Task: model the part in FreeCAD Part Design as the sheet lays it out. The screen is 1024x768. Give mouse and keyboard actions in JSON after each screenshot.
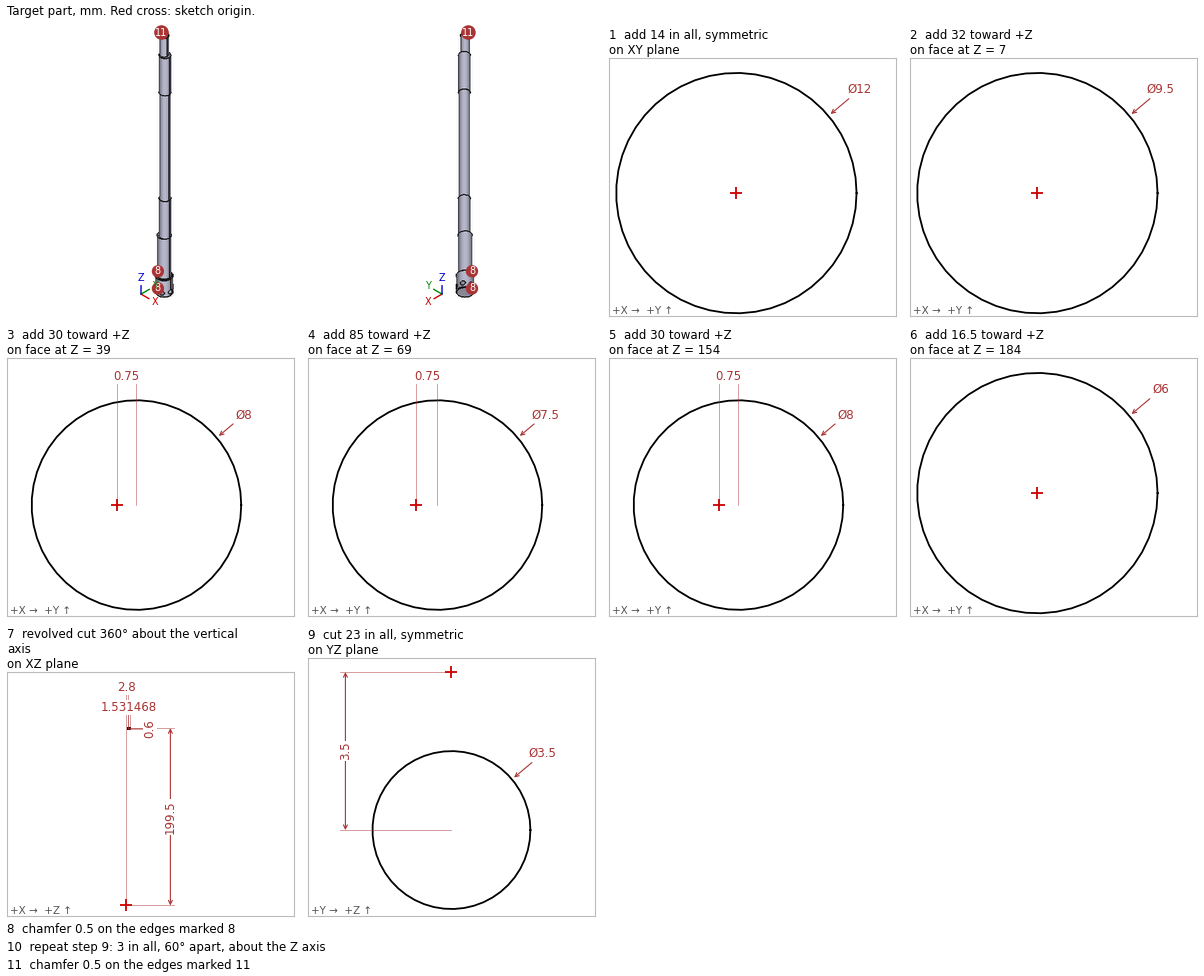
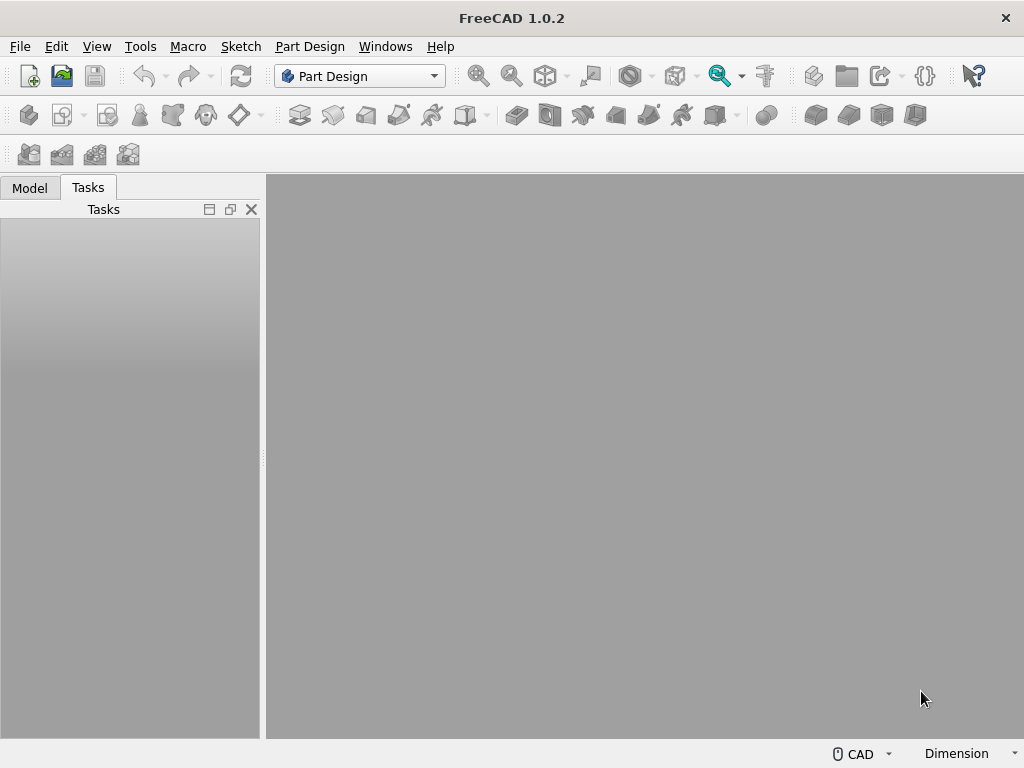
{"action": "left_click", "coordinate": [29, 76]}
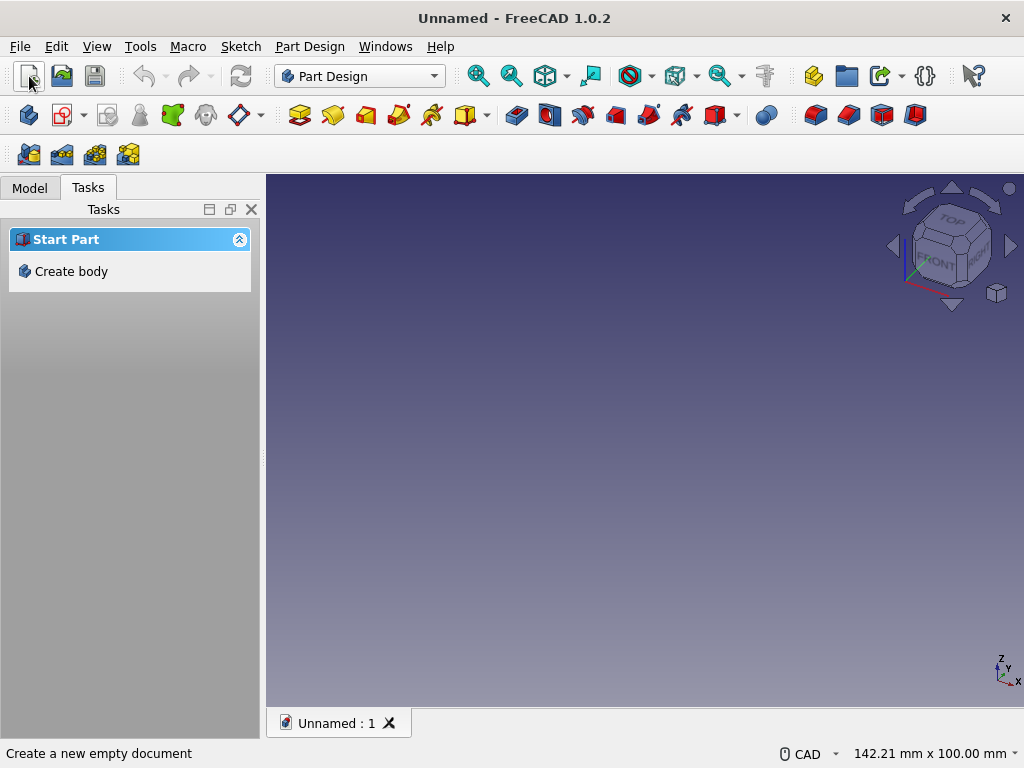
{"action": "left_click", "coordinate": [62, 116]}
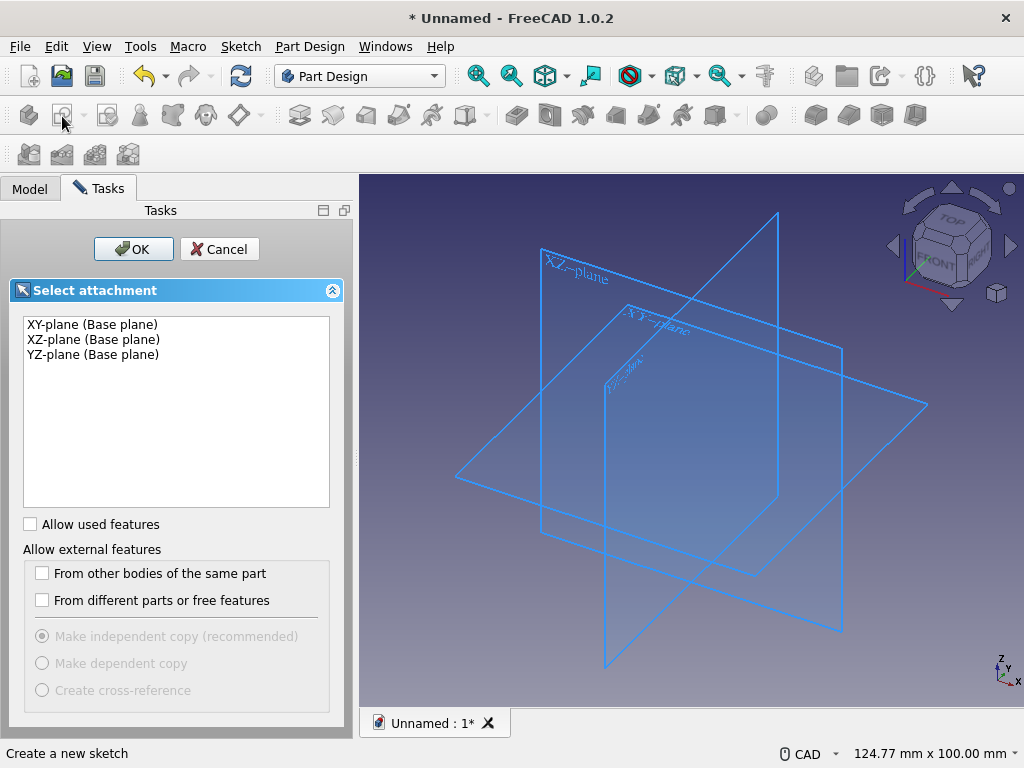
{"action": "left_click", "coordinate": [84, 324]}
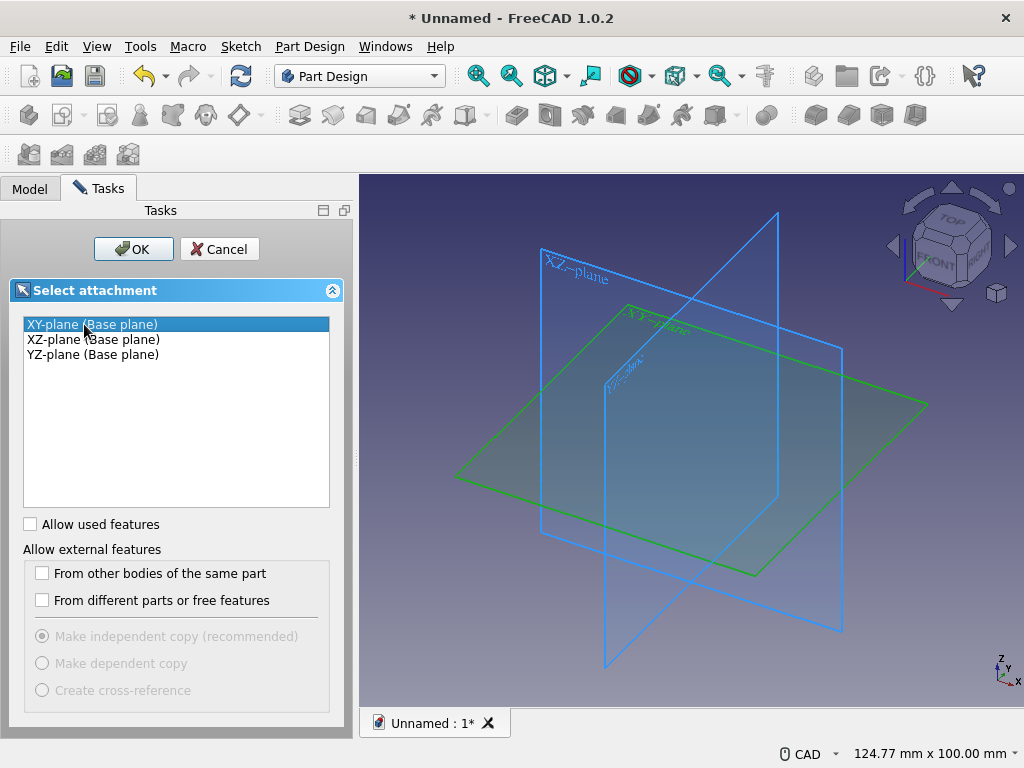
{"action": "left_click", "coordinate": [134, 249]}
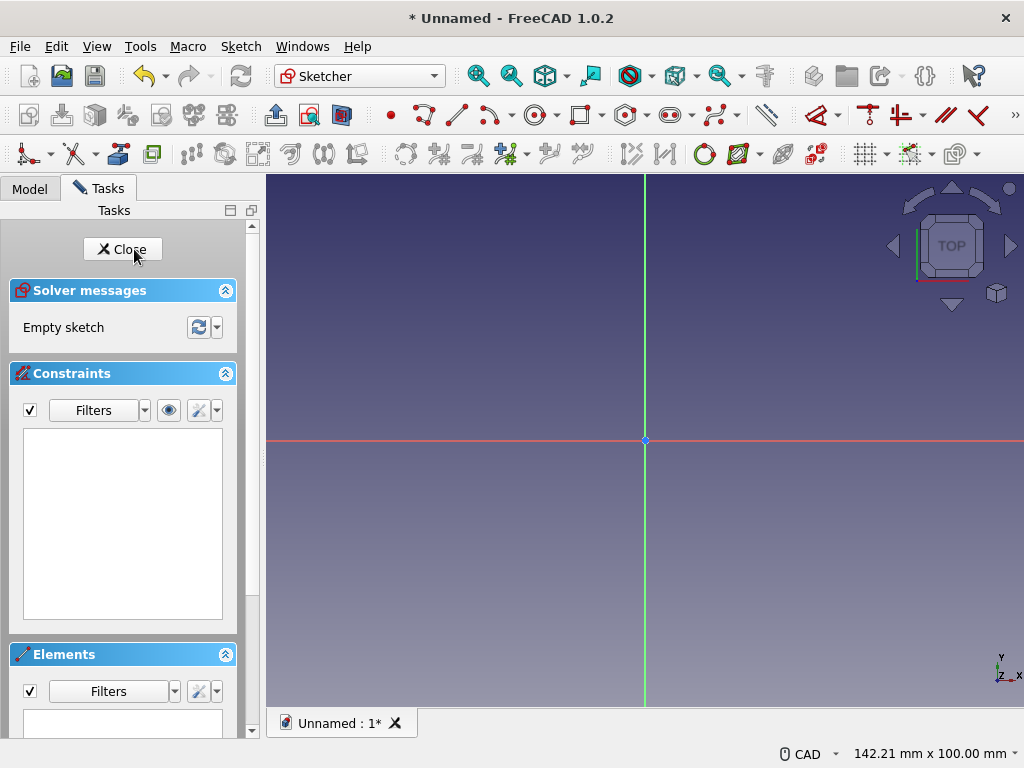
{"action": "scroll", "coordinate": [662, 440], "scroll_direction": "up", "scroll_amount": 8}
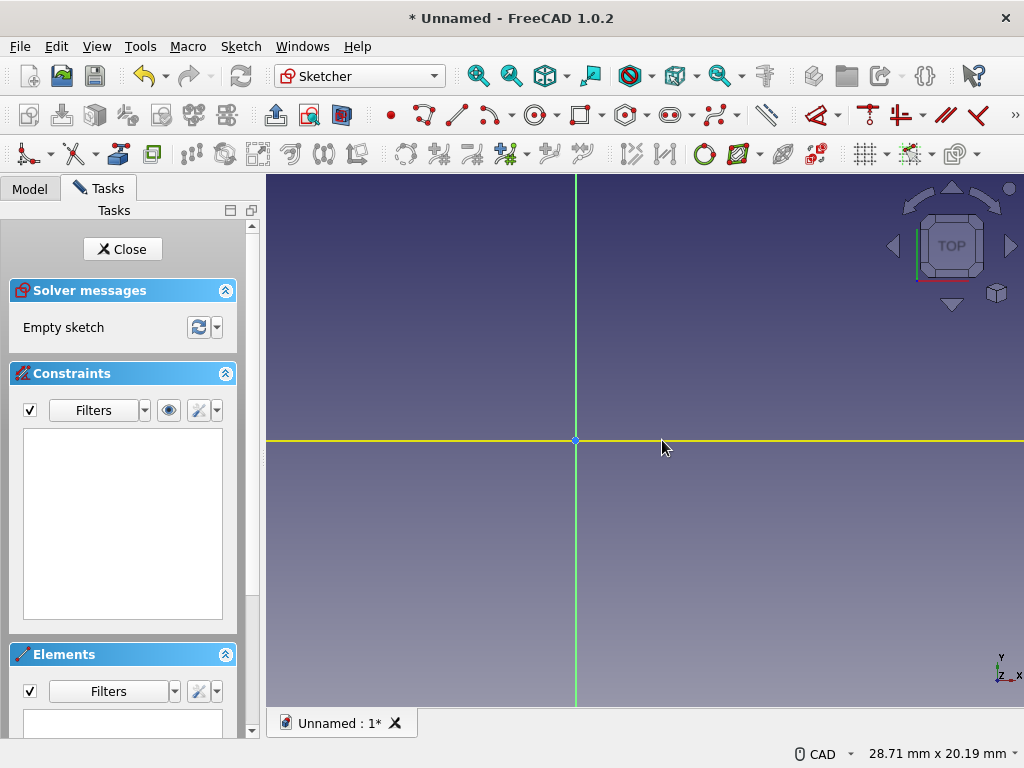
{"action": "left_click", "coordinate": [534, 116]}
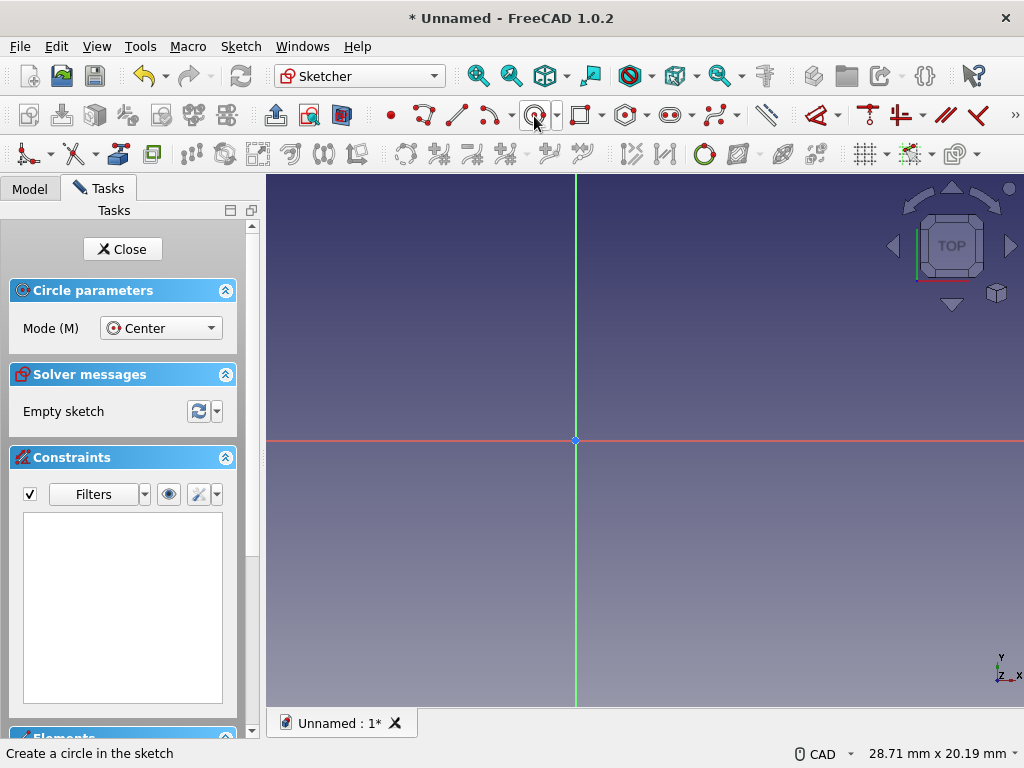
{"action": "left_click", "coordinate": [576, 440]}
{"action": "left_click", "coordinate": [688, 328]}
{"action": "key", "text": "Escape"}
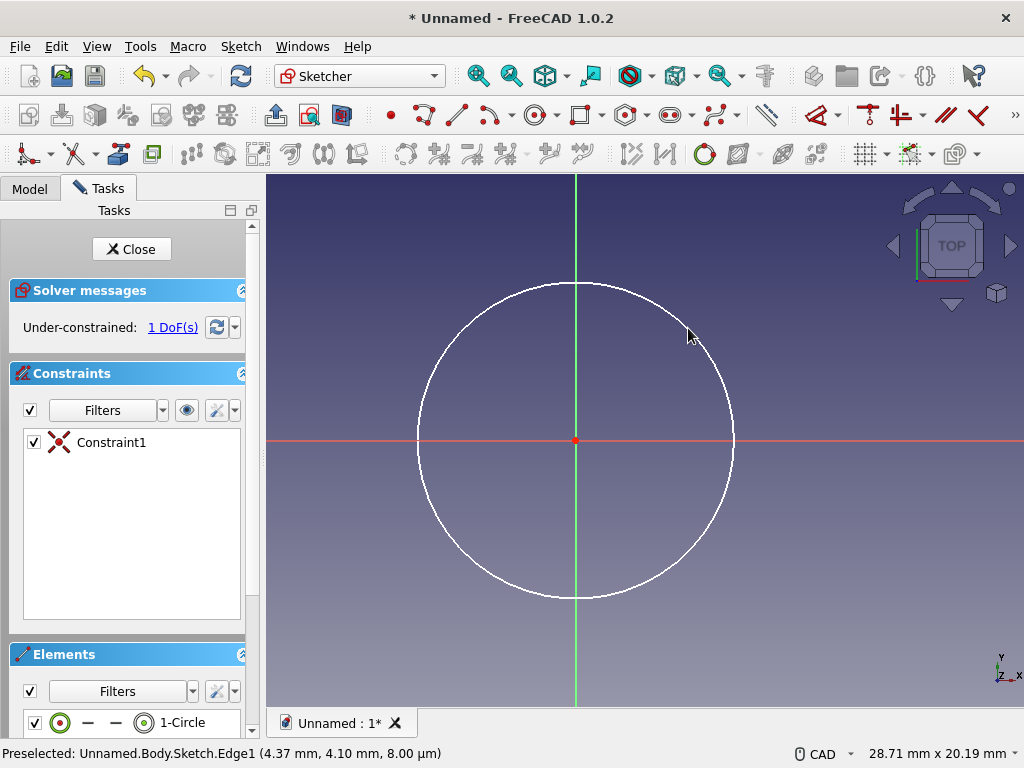
{"action": "left_click", "coordinate": [687, 328]}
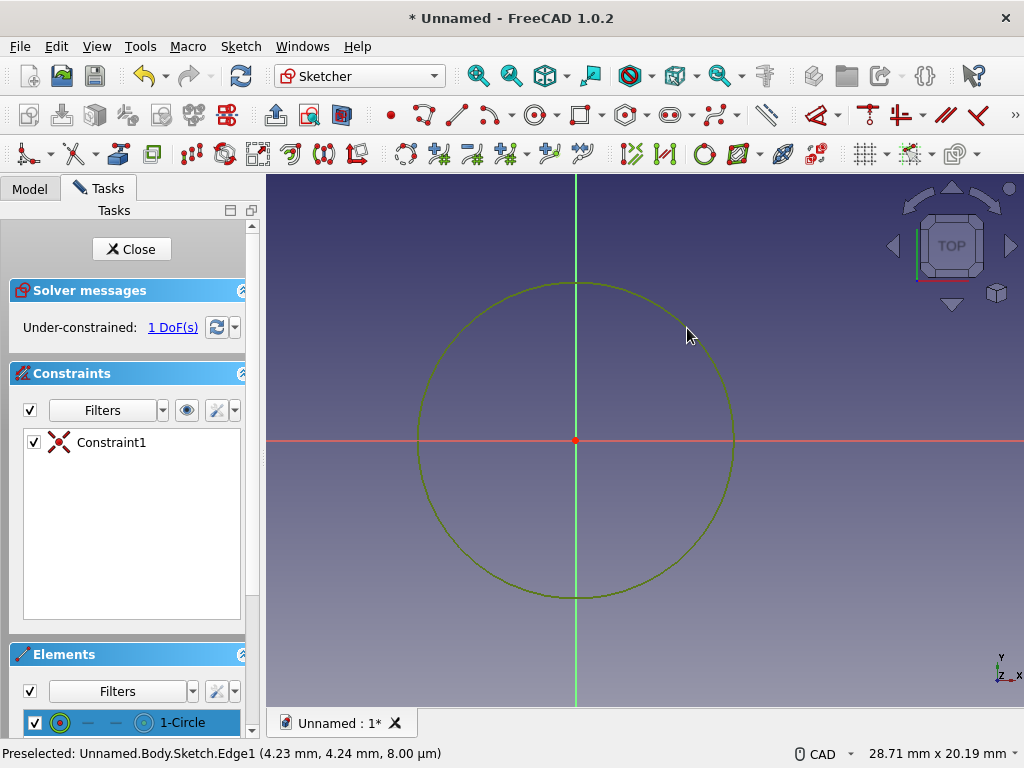
{"action": "left_click", "coordinate": [838, 116]}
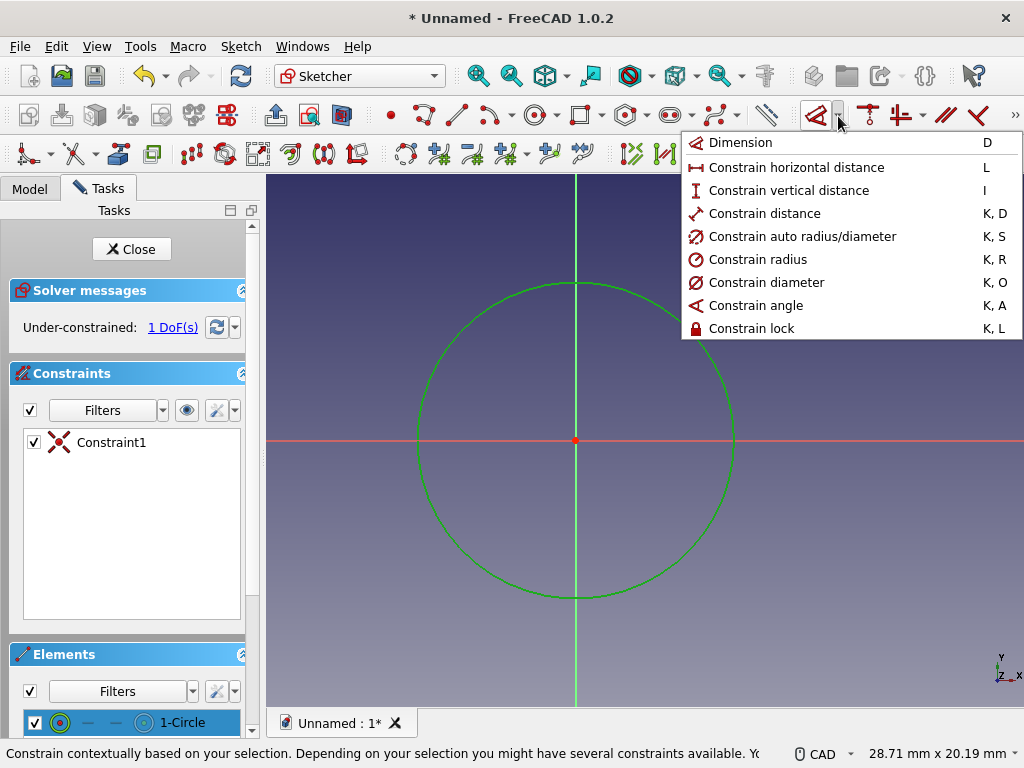
{"action": "left_click", "coordinate": [852, 282]}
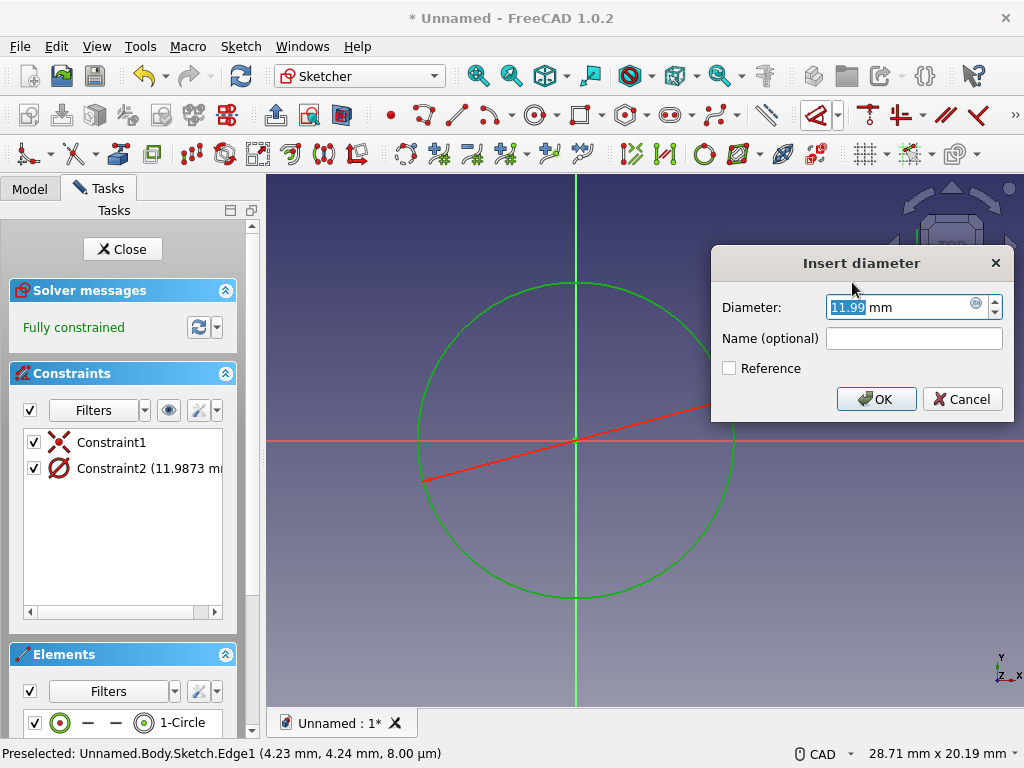
{"action": "type", "text": "12"}
{"action": "key", "text": "Return"}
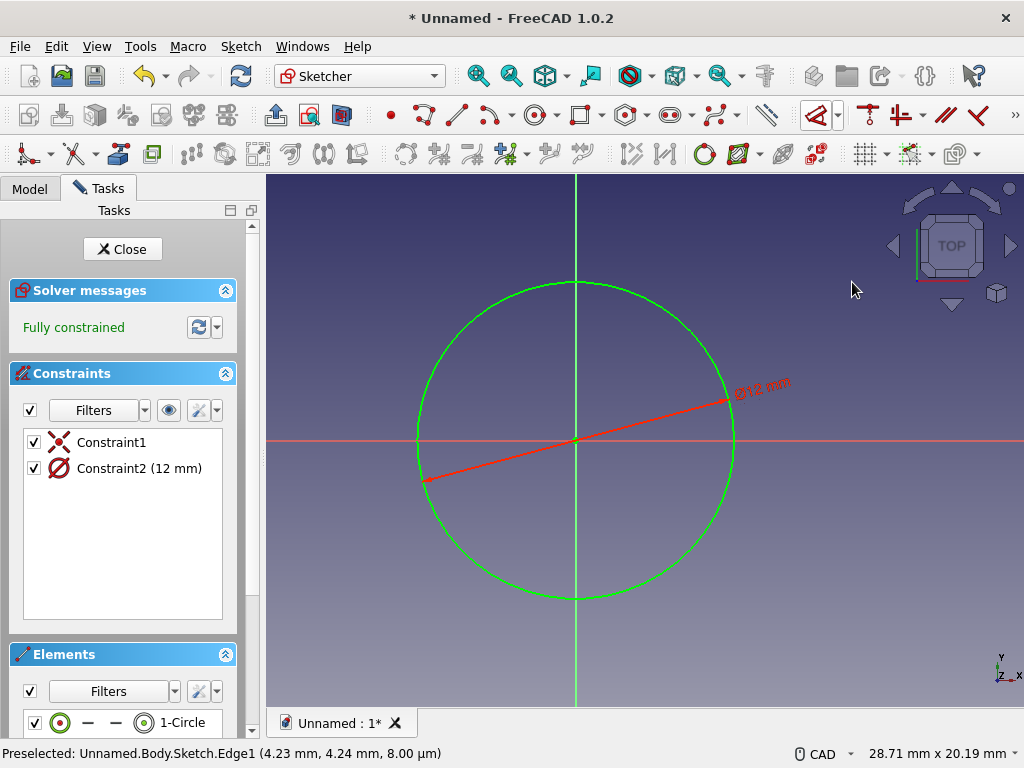
{"action": "left_click", "coordinate": [123, 249]}